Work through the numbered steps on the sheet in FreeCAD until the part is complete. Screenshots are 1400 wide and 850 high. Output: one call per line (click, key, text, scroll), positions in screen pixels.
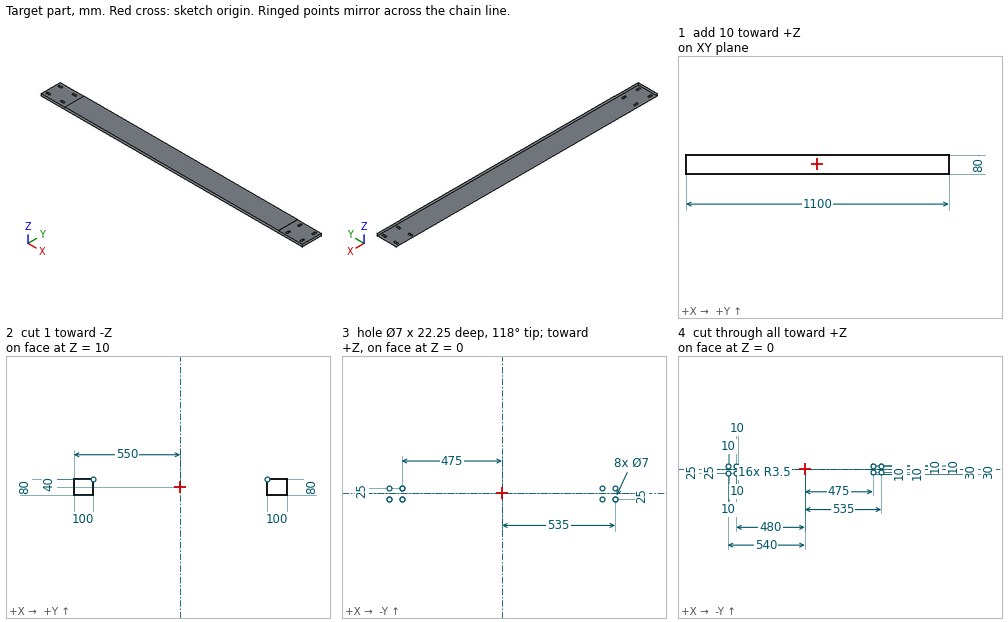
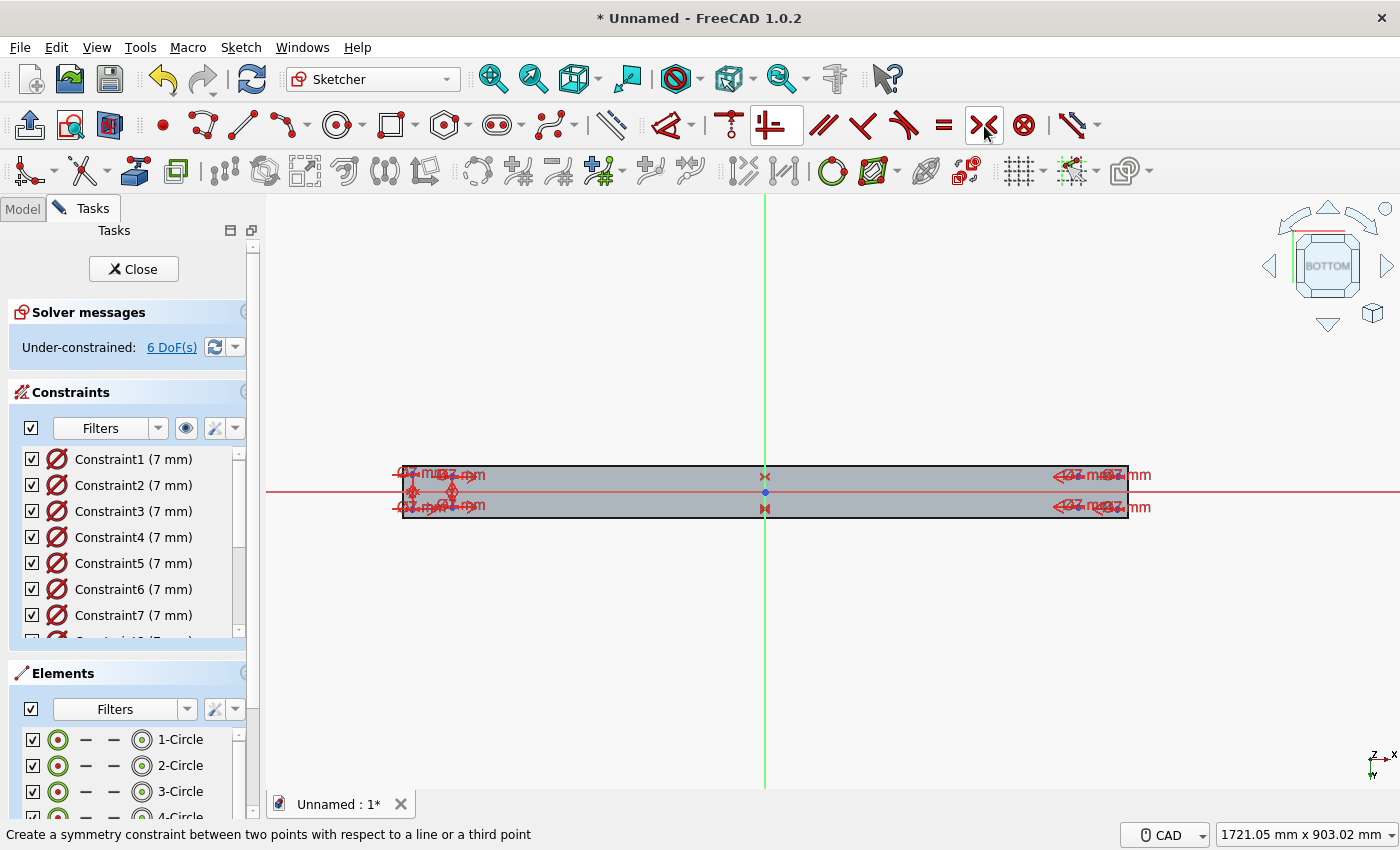
click(1118, 509)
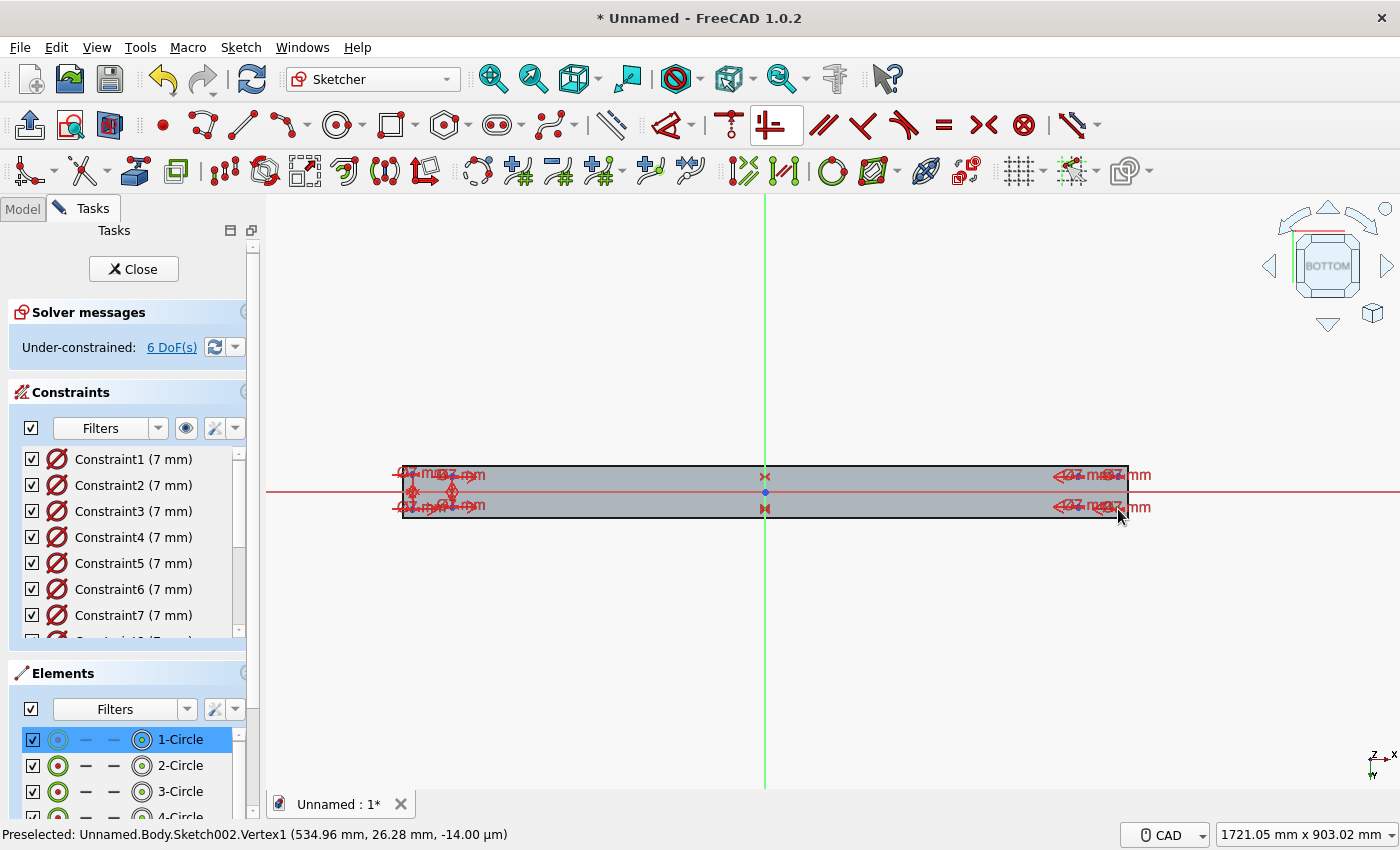
click(1118, 477)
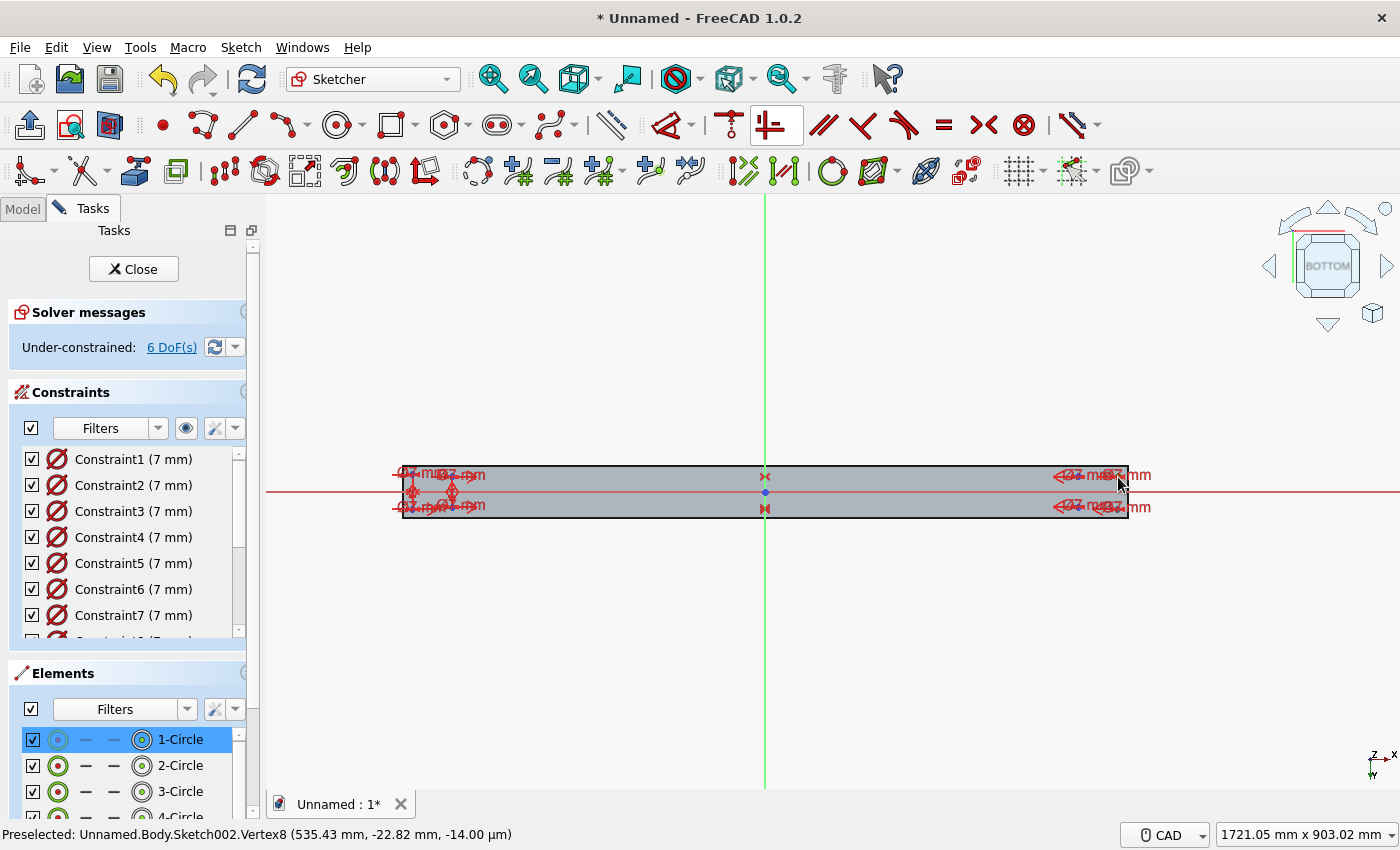
click(361, 492)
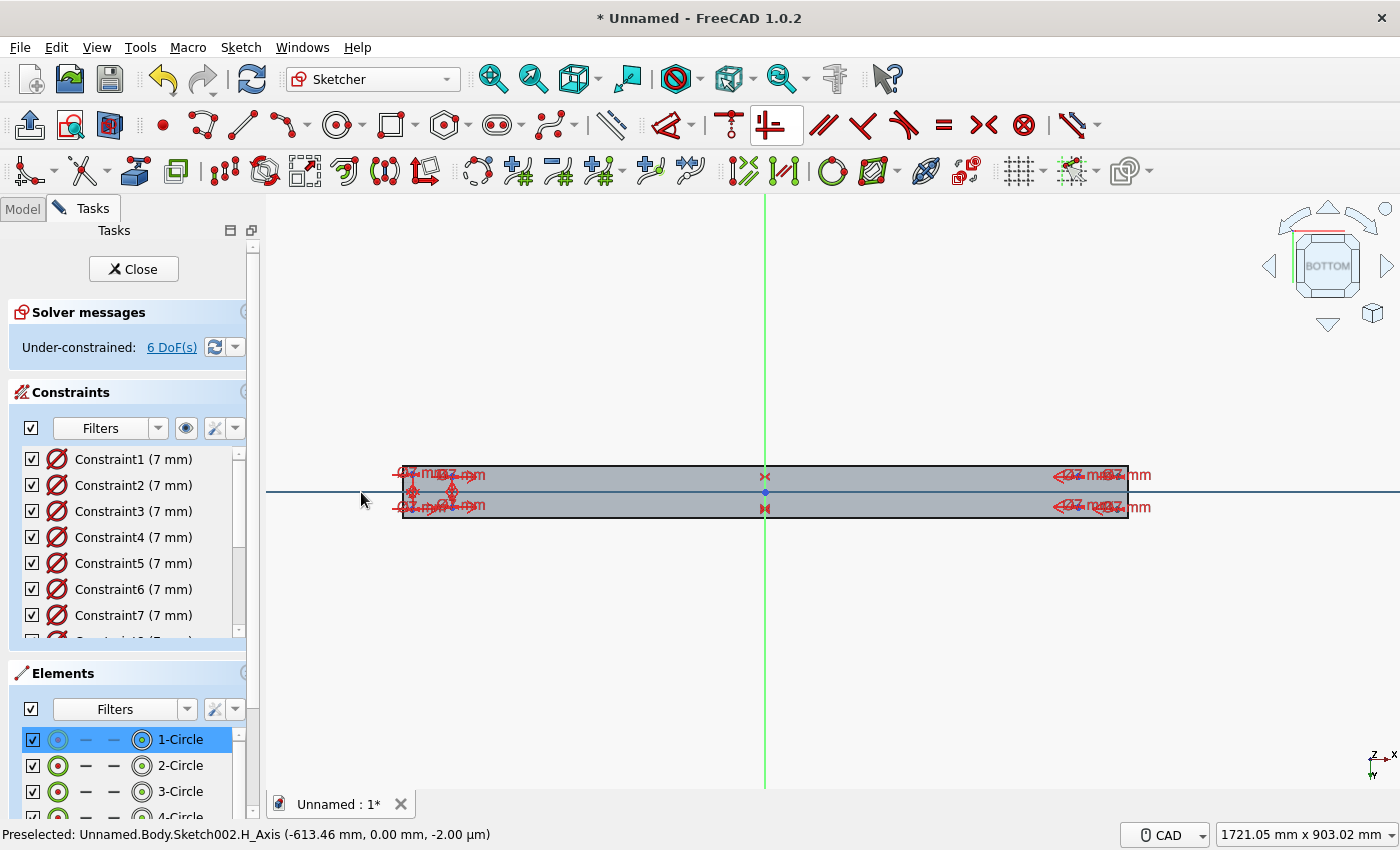
click(984, 126)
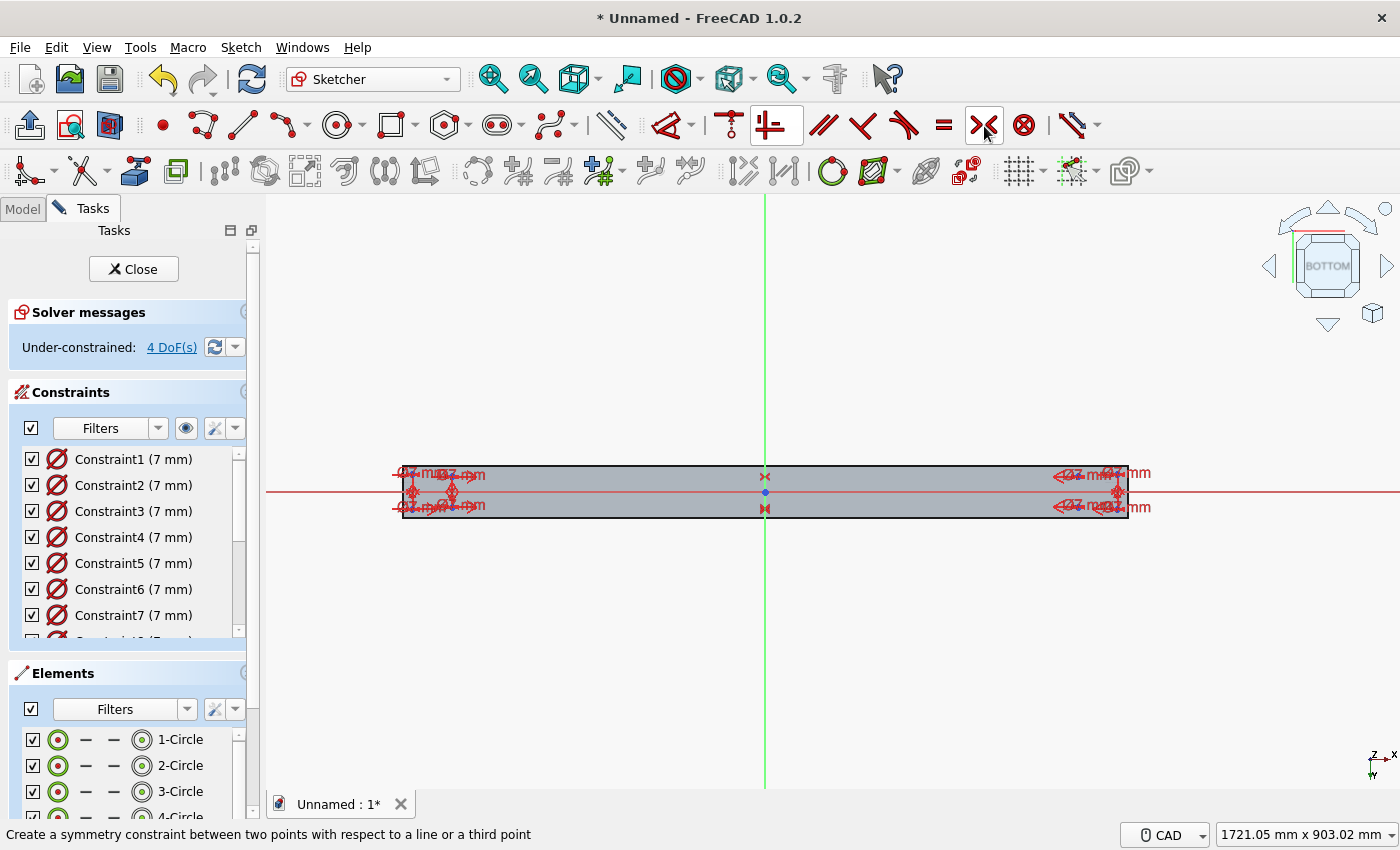
key(d)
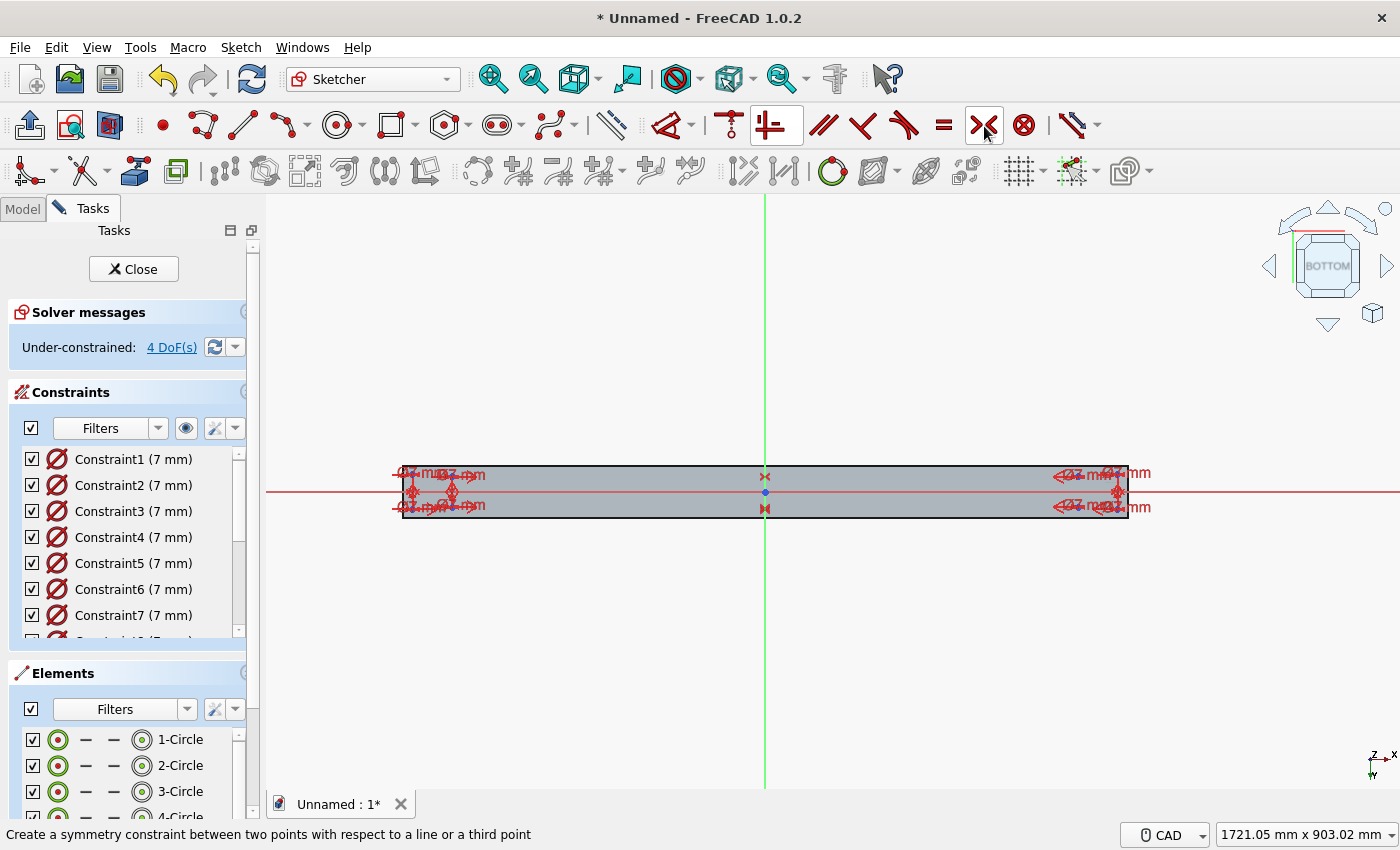
scroll(1118, 509, up, 5)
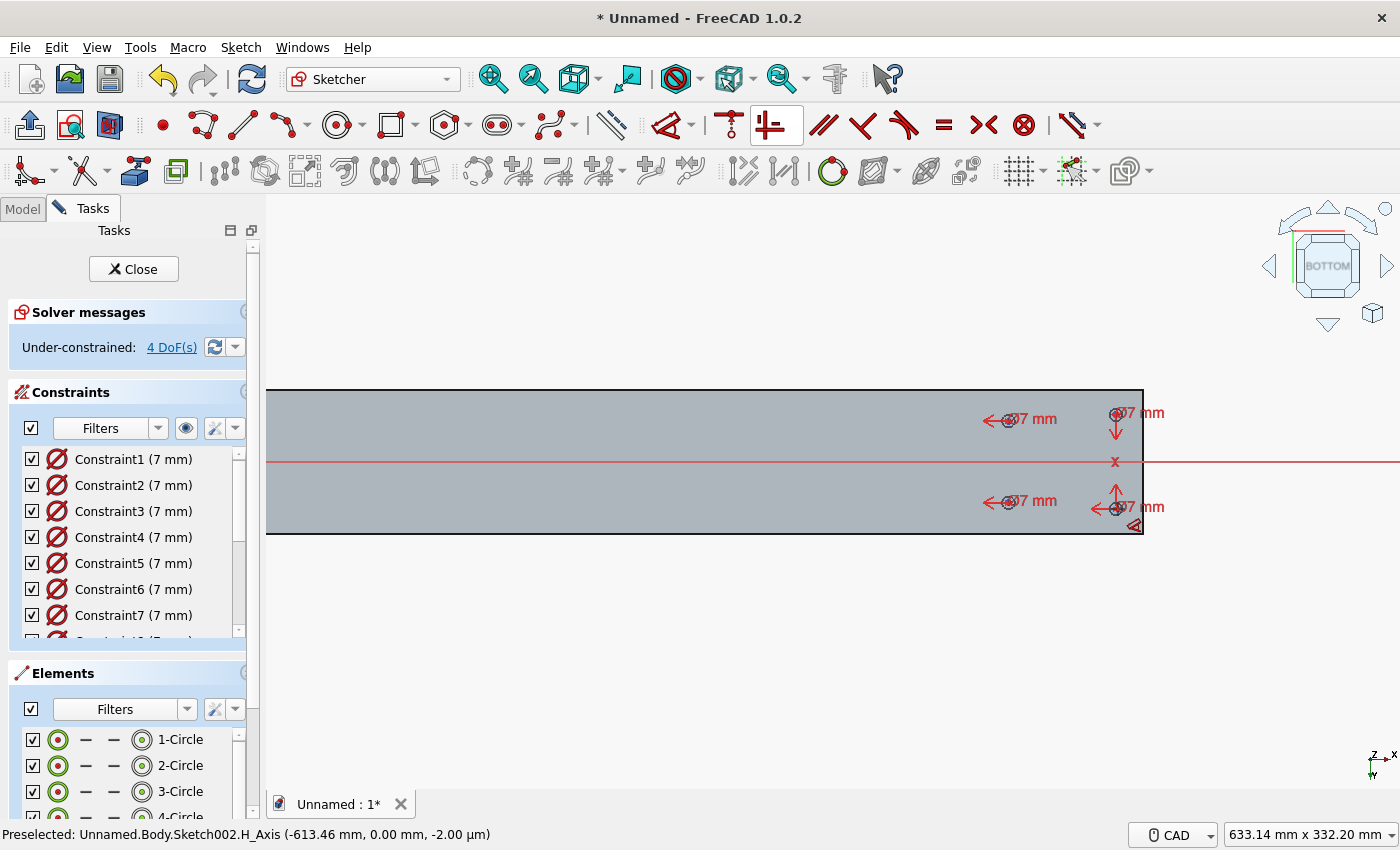
click(1116, 509)
click(1150, 486)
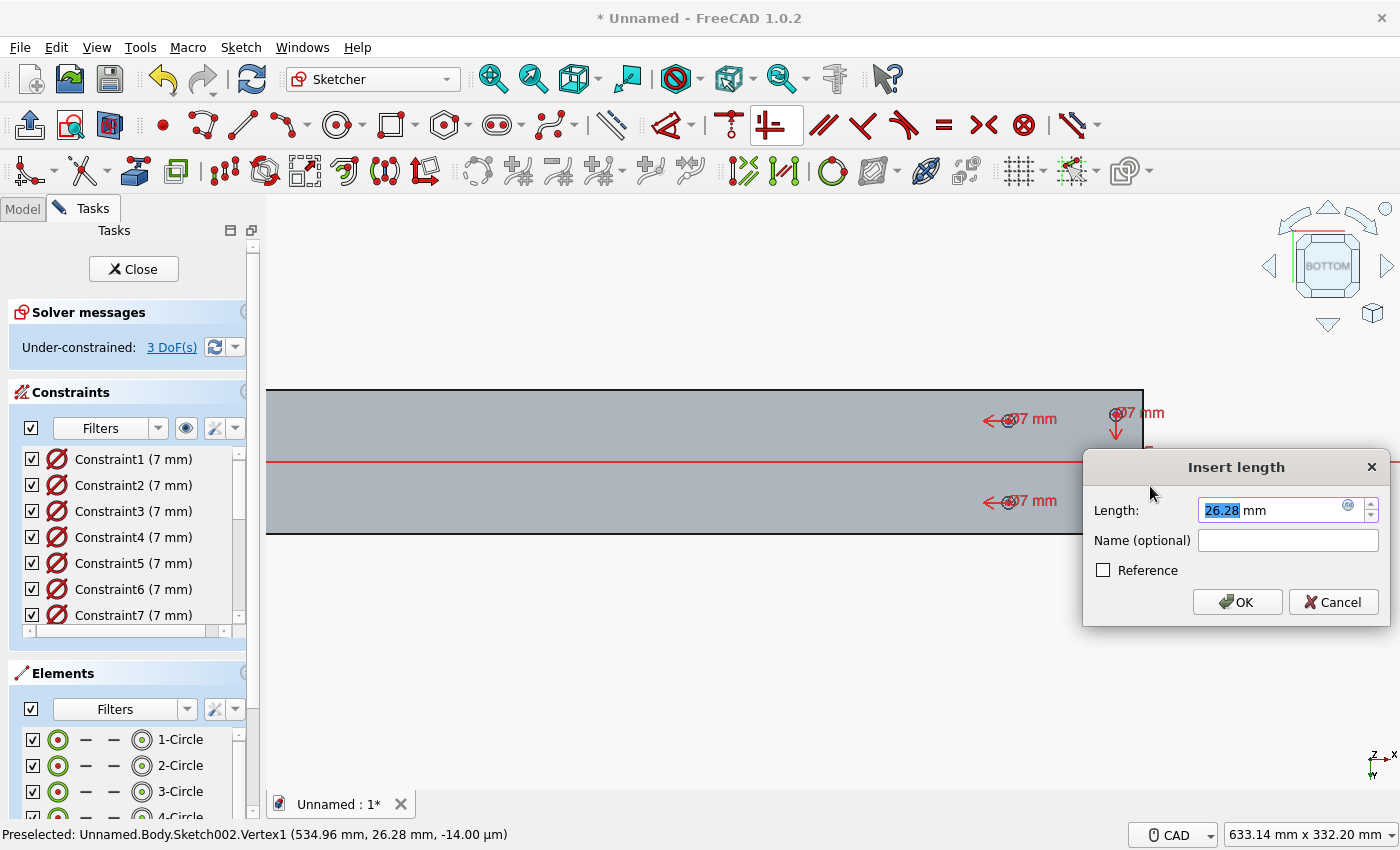
text(25)
key(Return)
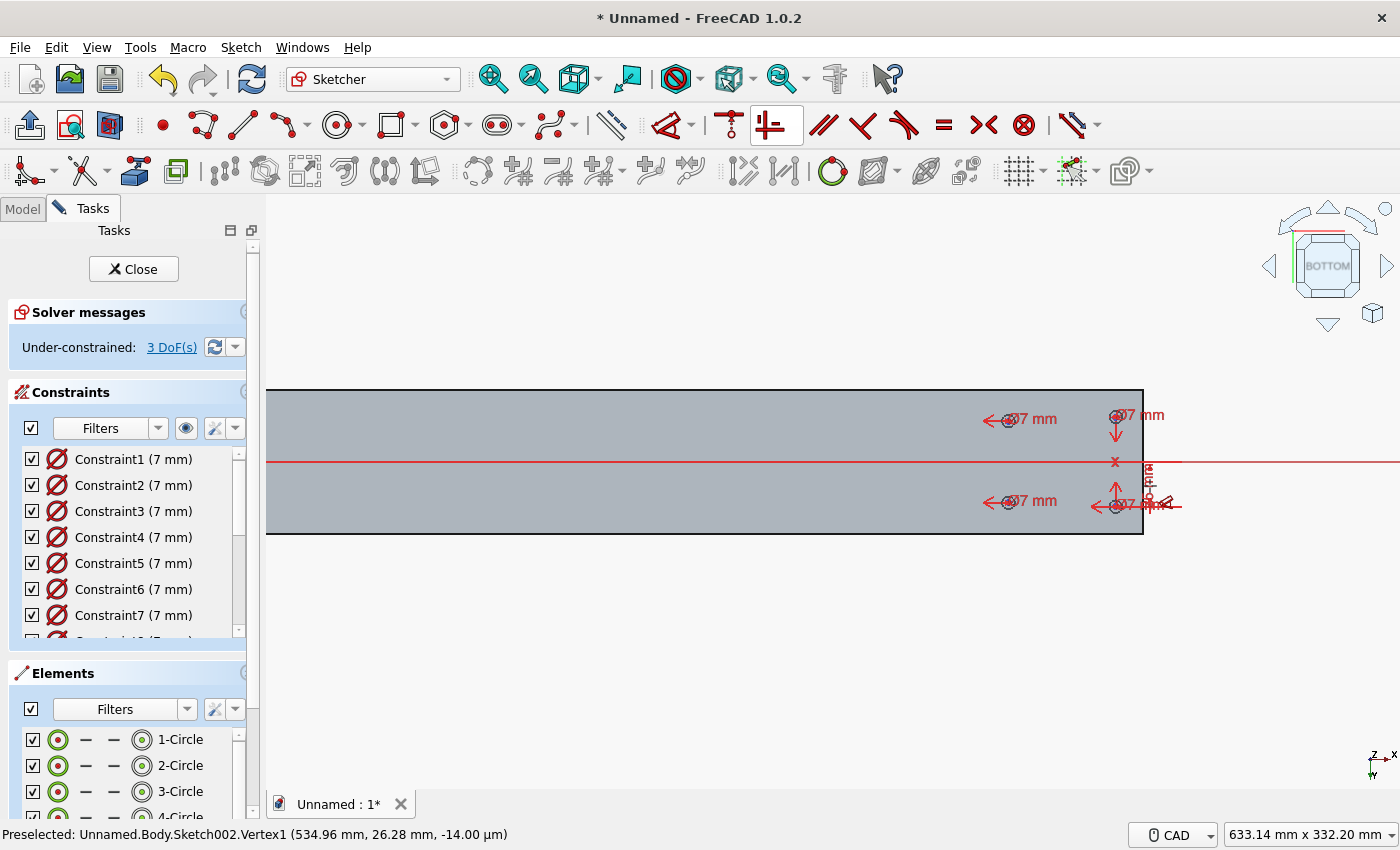
scroll(1118, 509, down, 5)